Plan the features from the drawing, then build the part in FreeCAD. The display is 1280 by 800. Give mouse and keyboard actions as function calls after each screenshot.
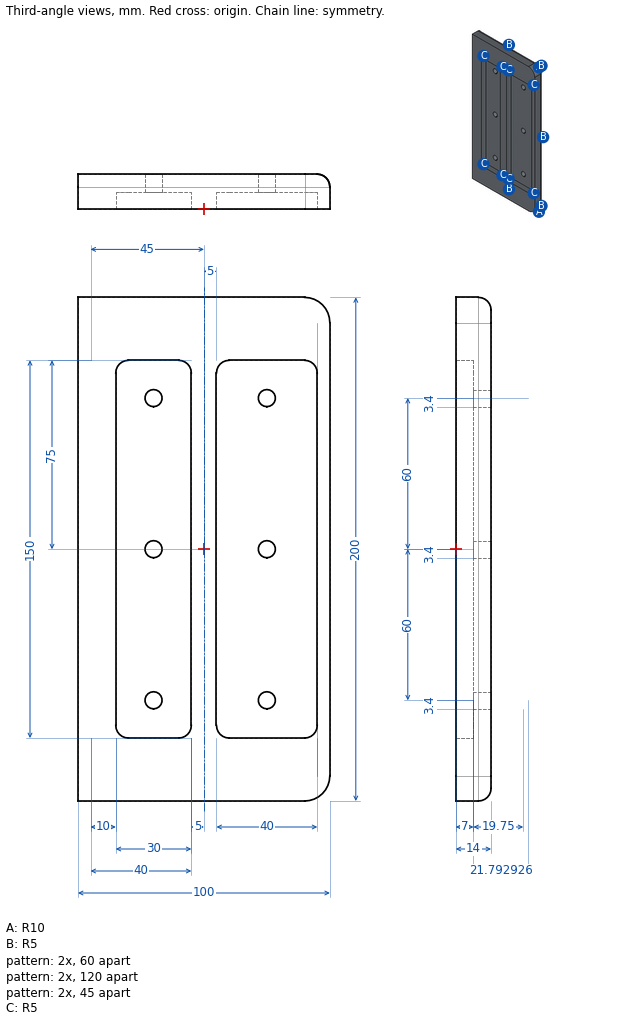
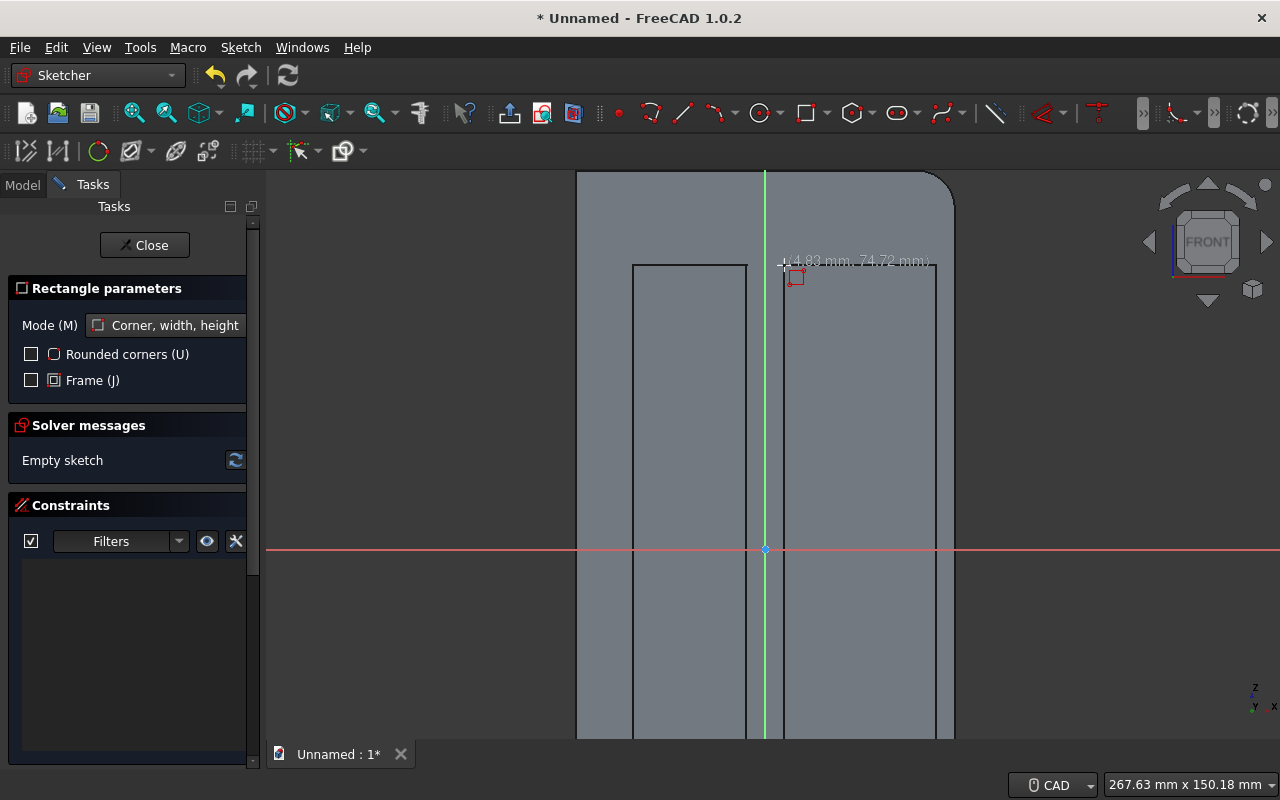
click(784, 265)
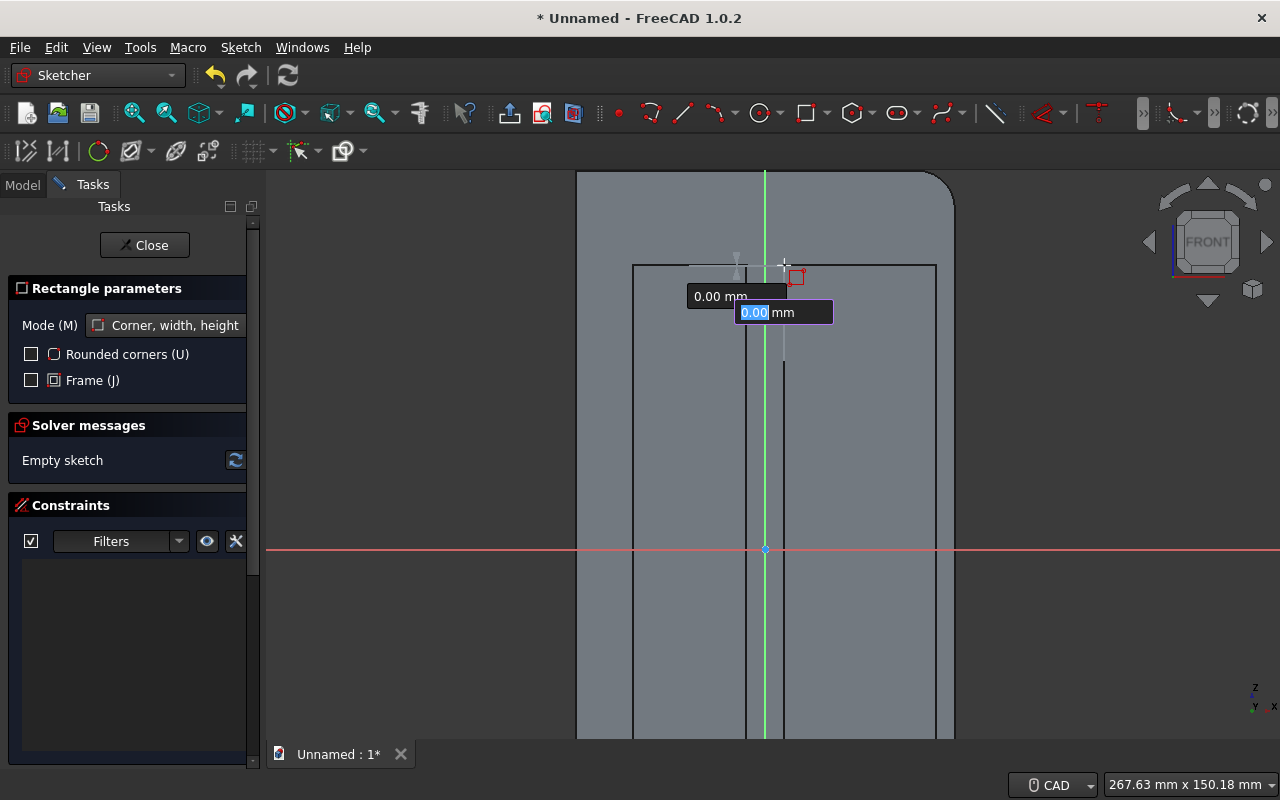
scroll(542, 261, down, 2)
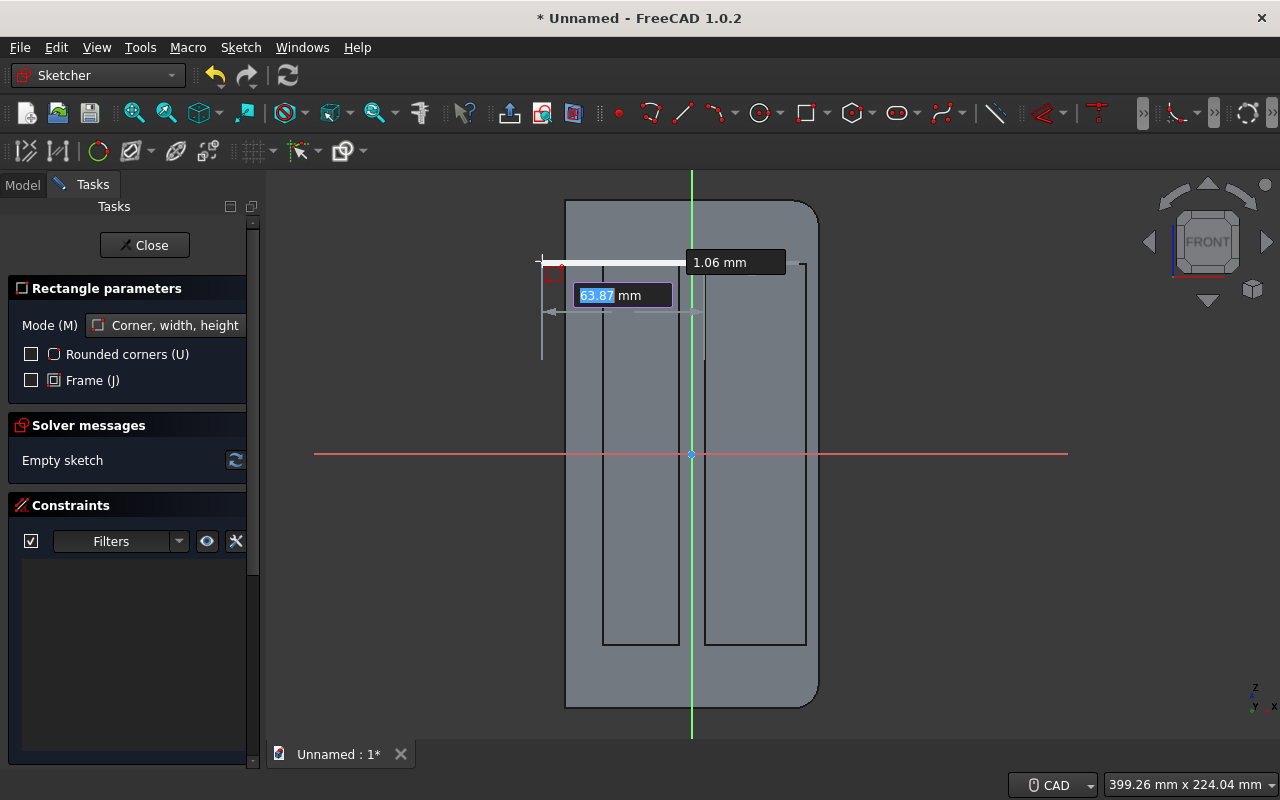
click(806, 645)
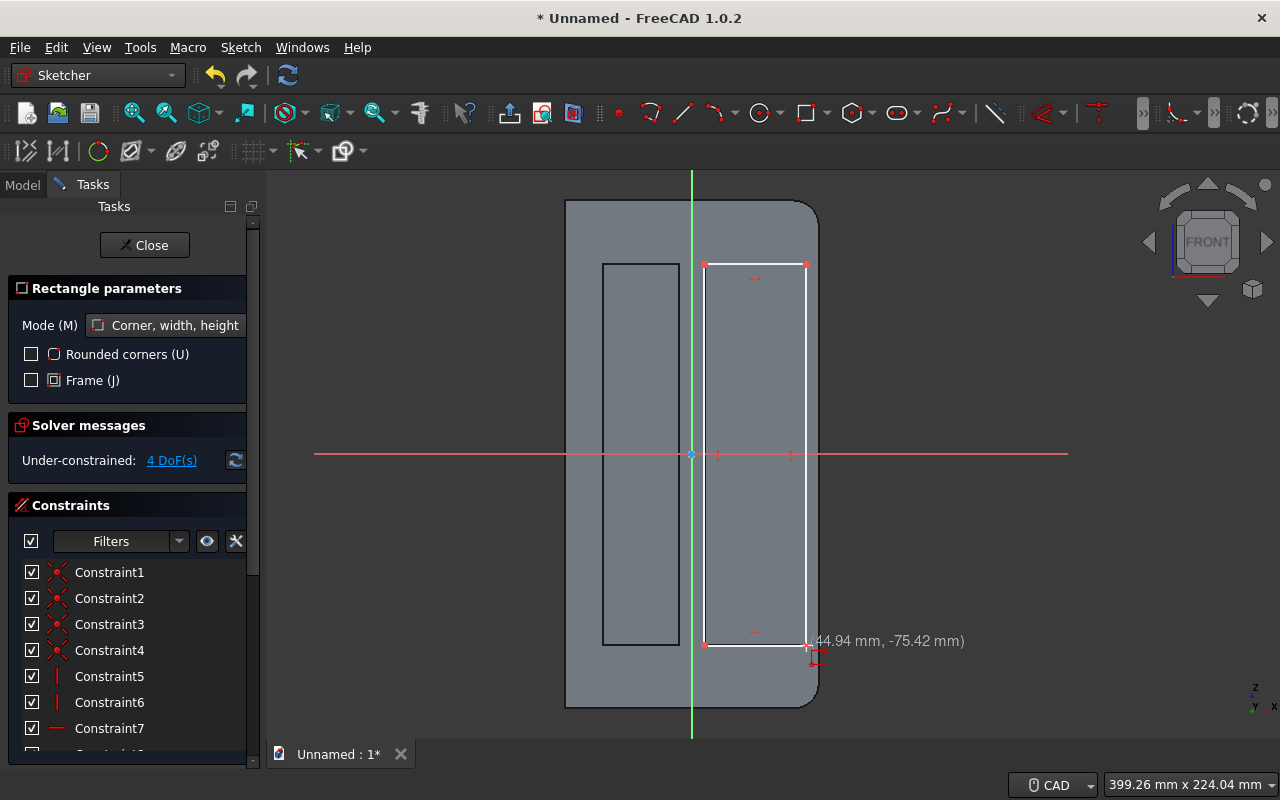
click(603, 264)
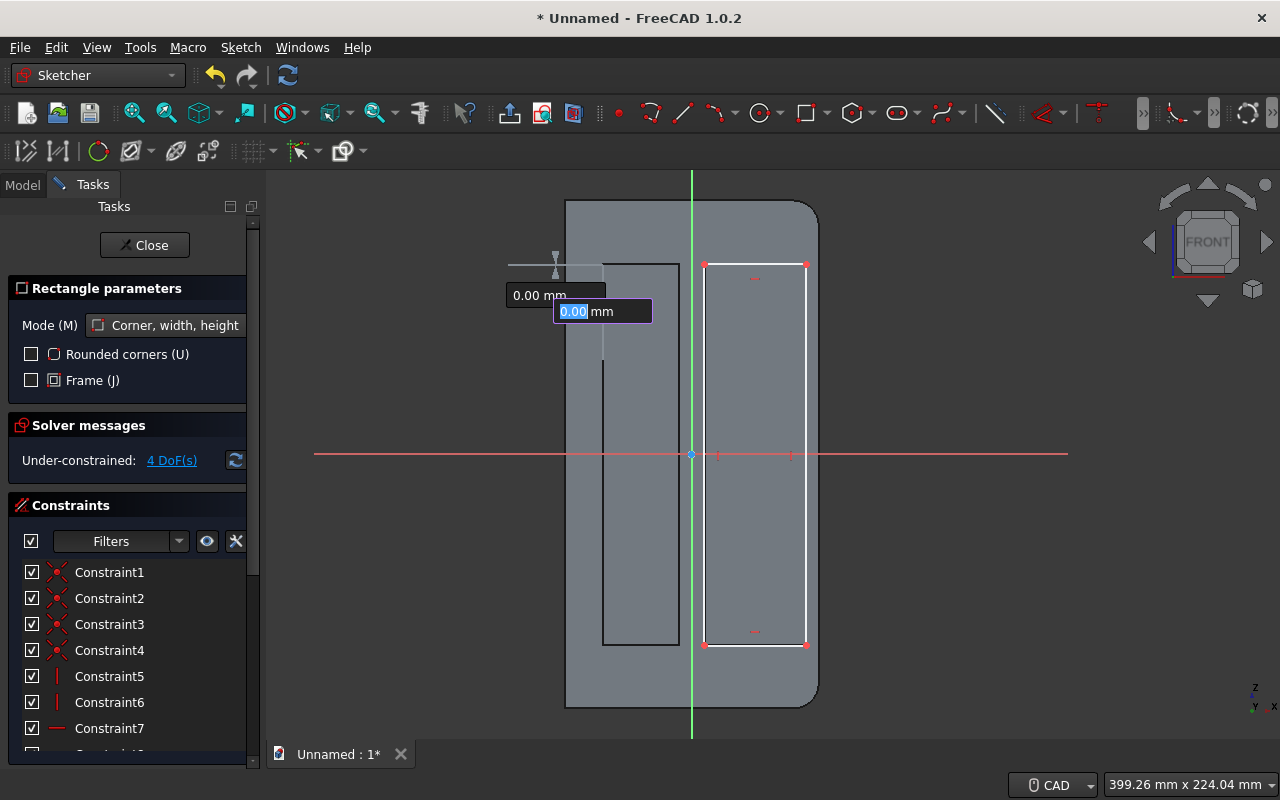
scroll(679, 645, up, 2)
move(679, 644)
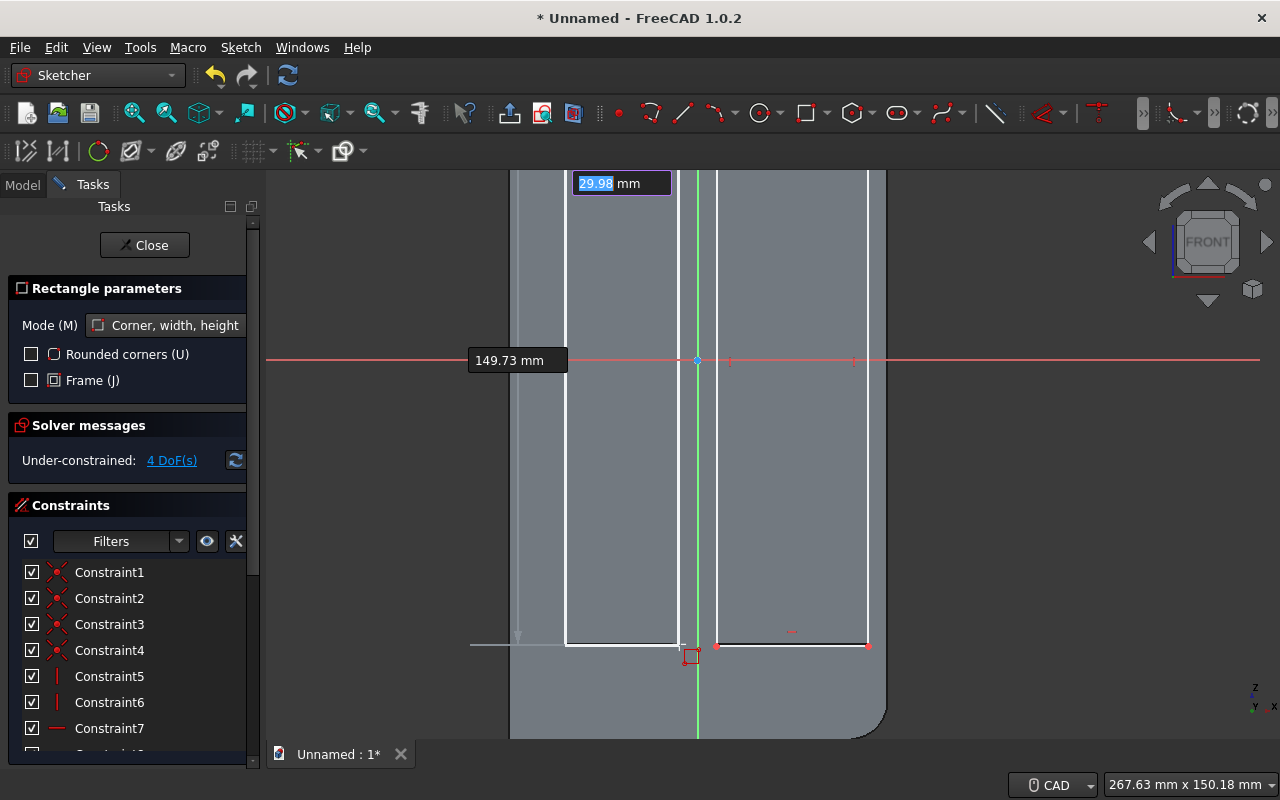
text(30)
key(Tab)
text(150)
key(Return)
key(Escape)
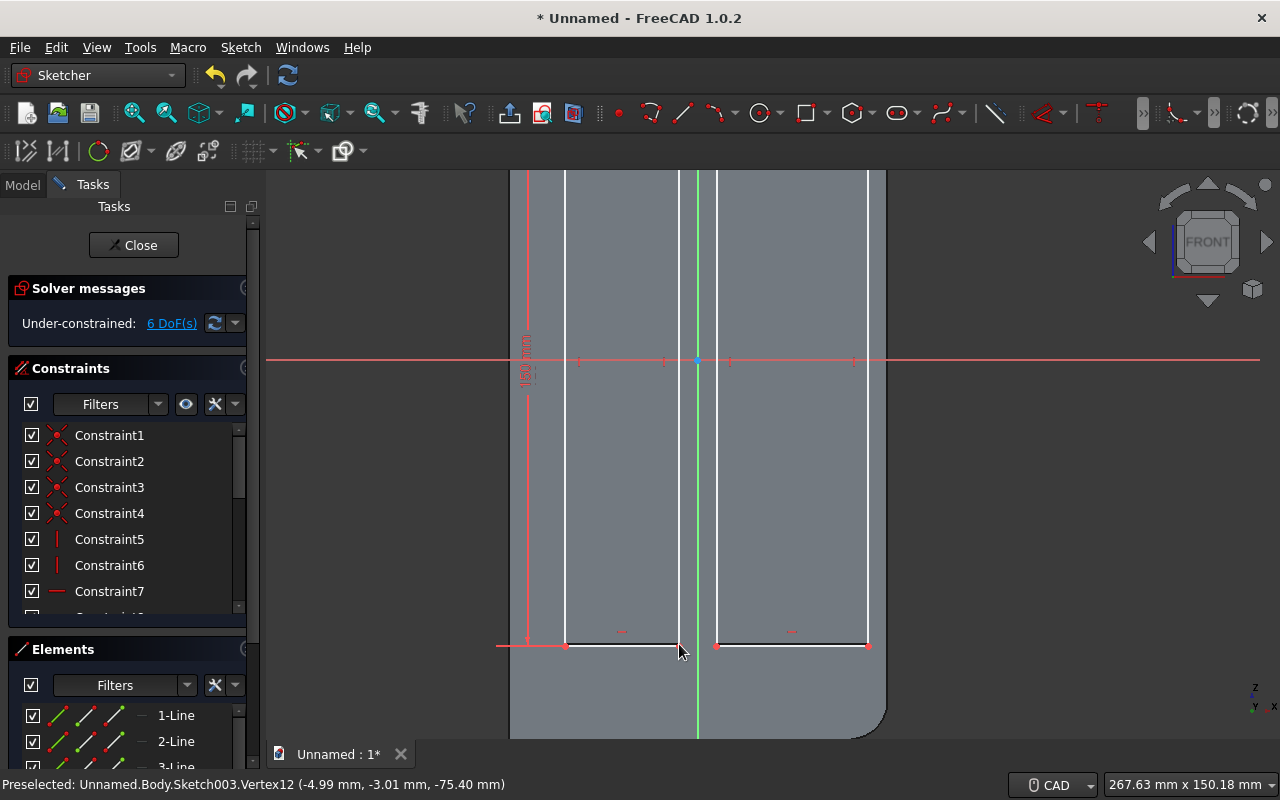
click(717, 646)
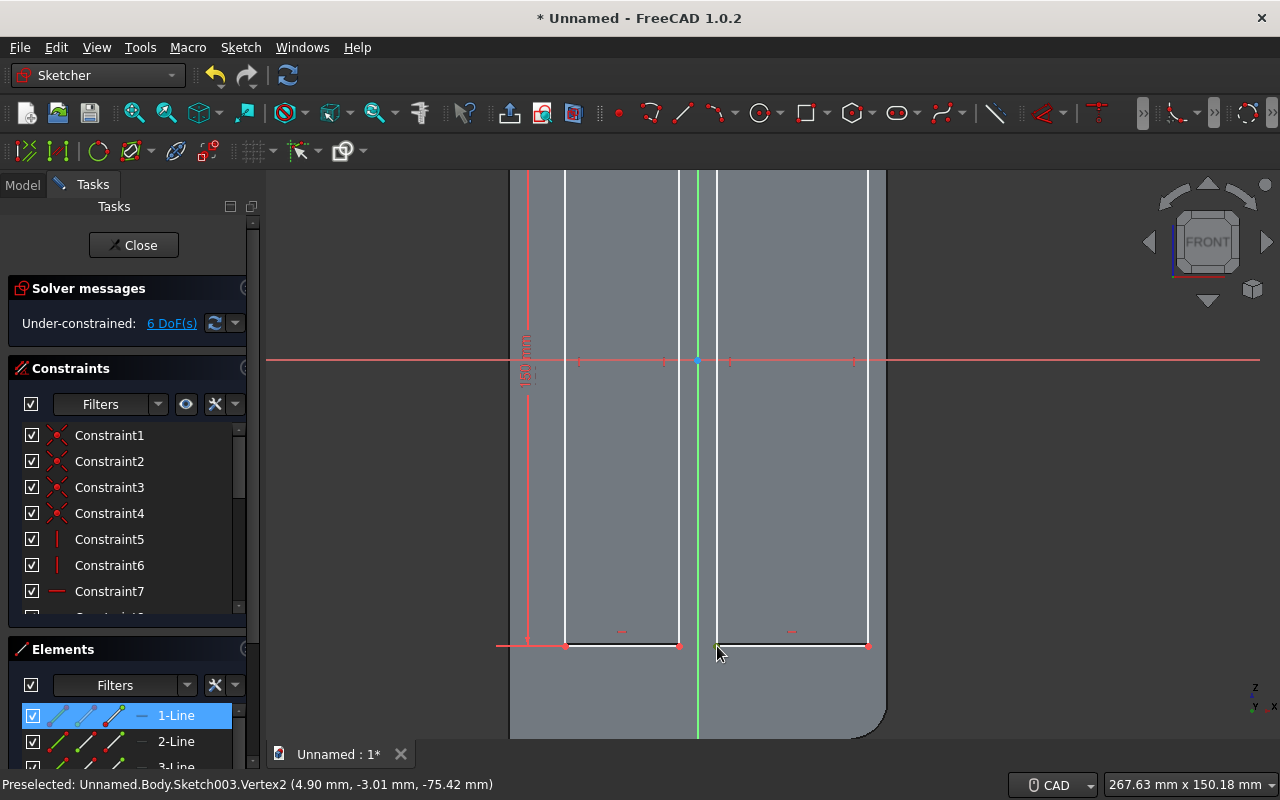
click(679, 646)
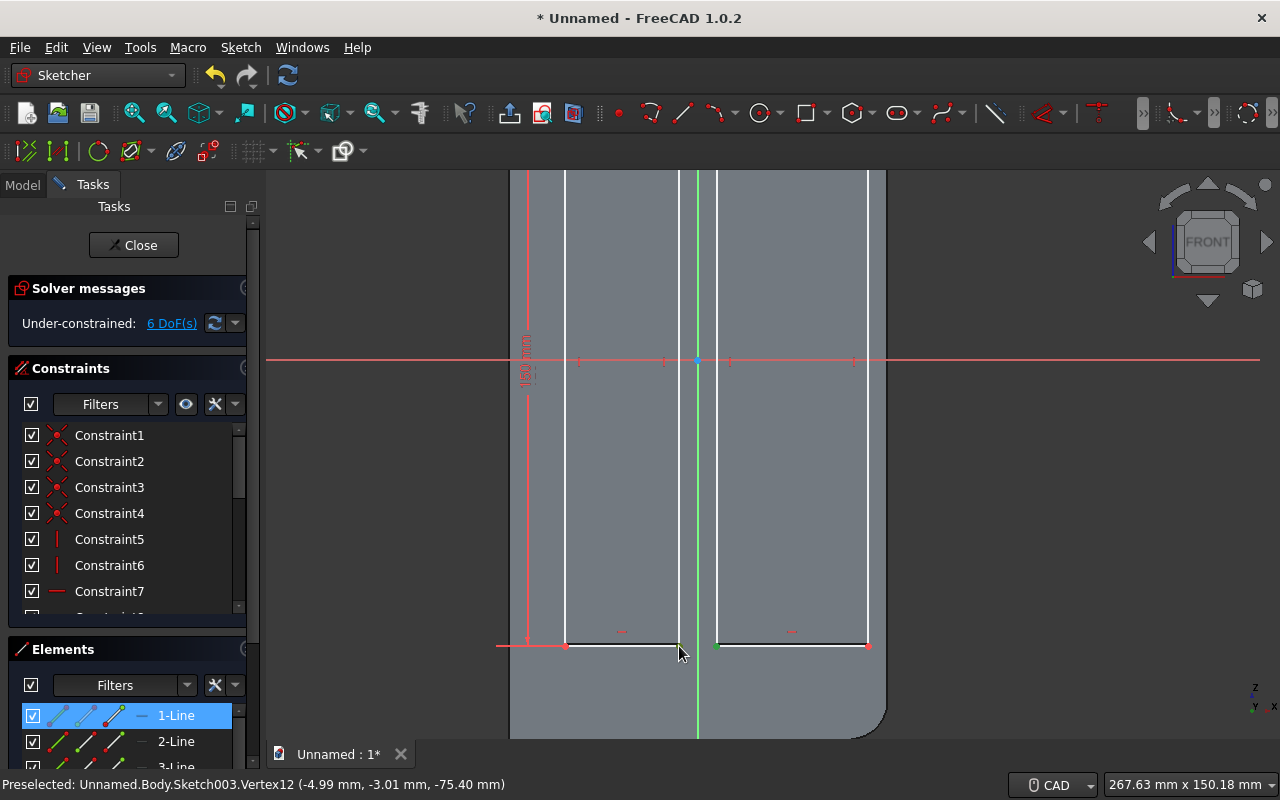
click(698, 674)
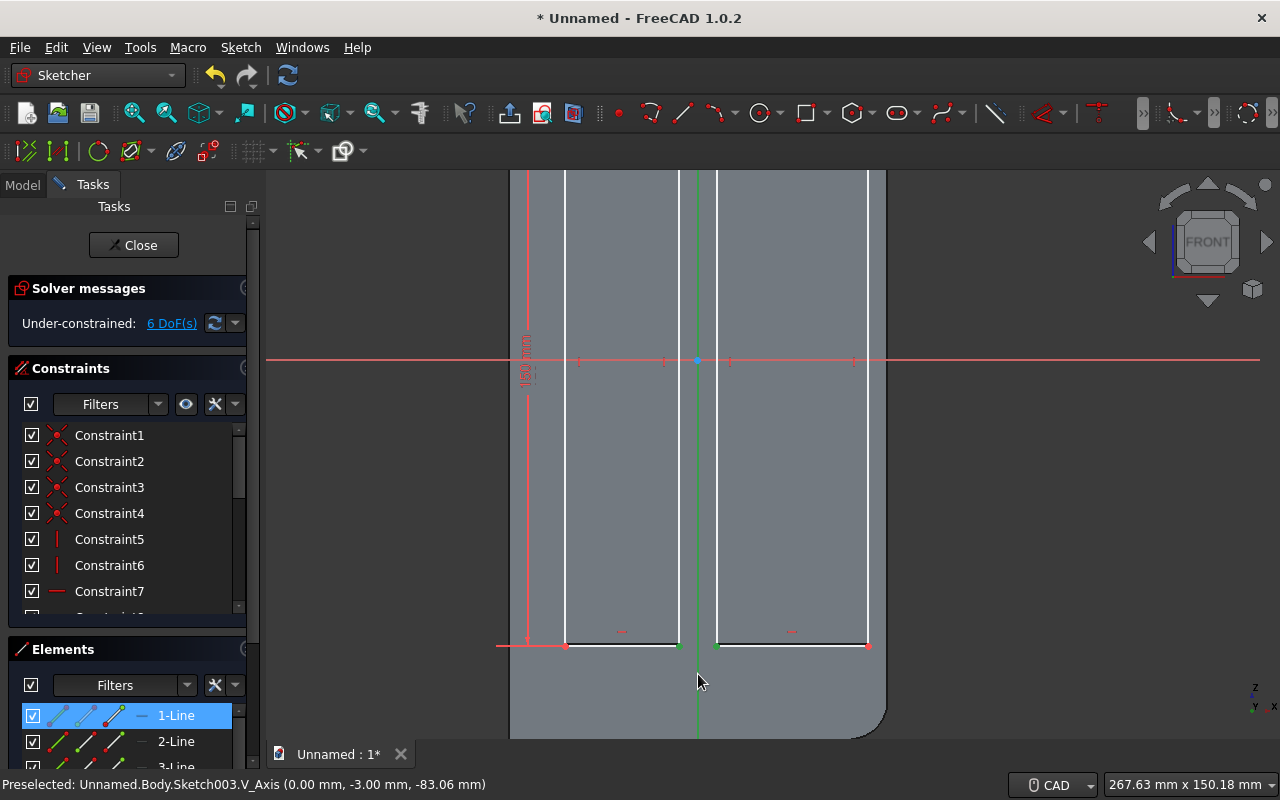
key(s)